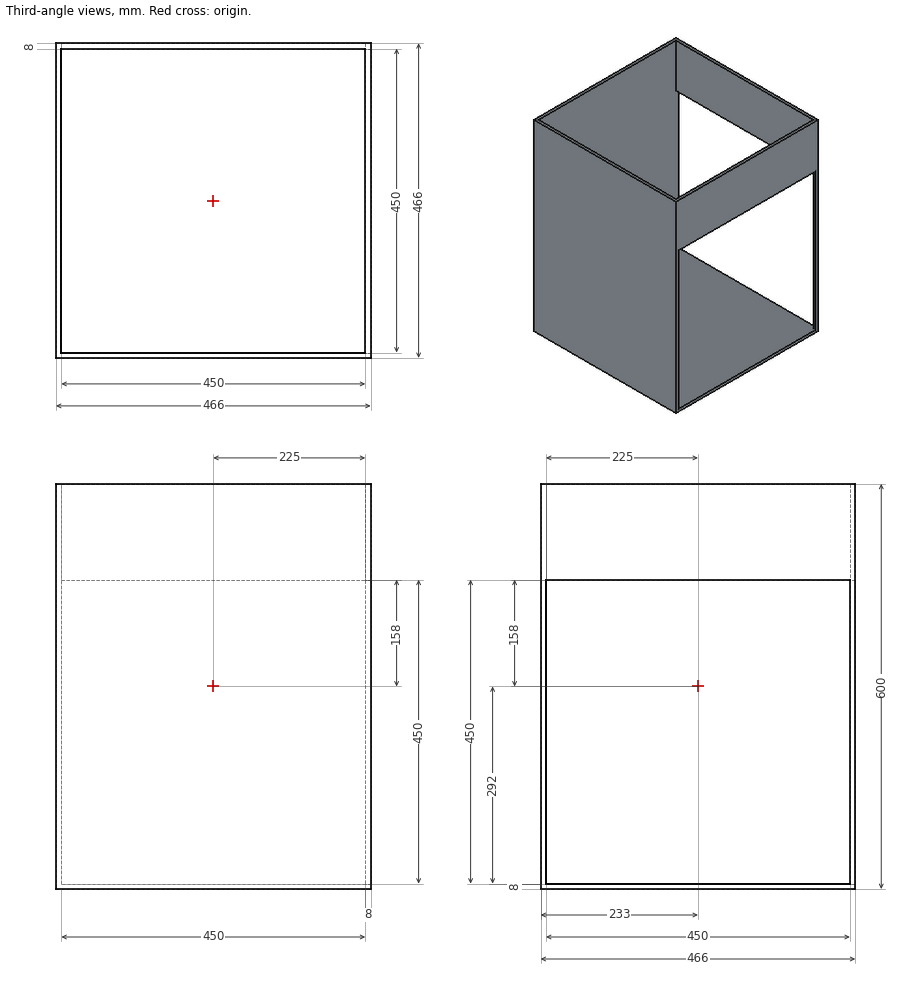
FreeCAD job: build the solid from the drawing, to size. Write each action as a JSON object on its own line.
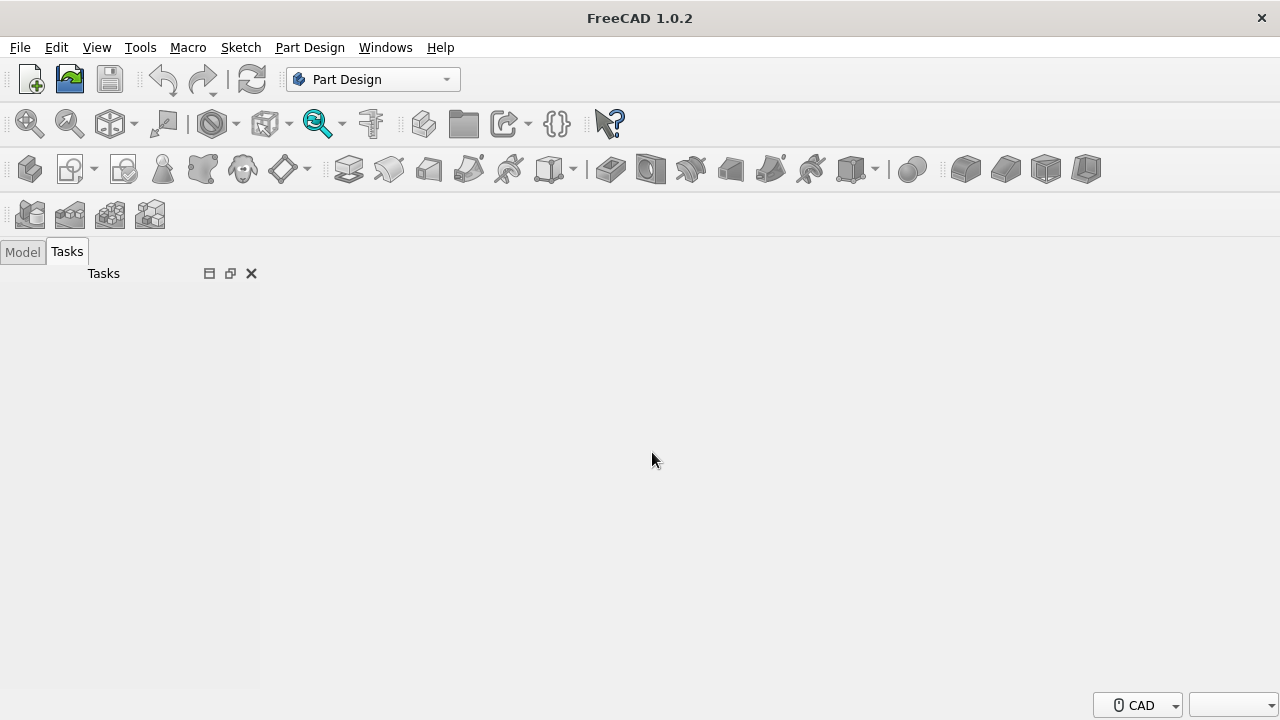
{"action": "left_click", "coordinate": [30, 80]}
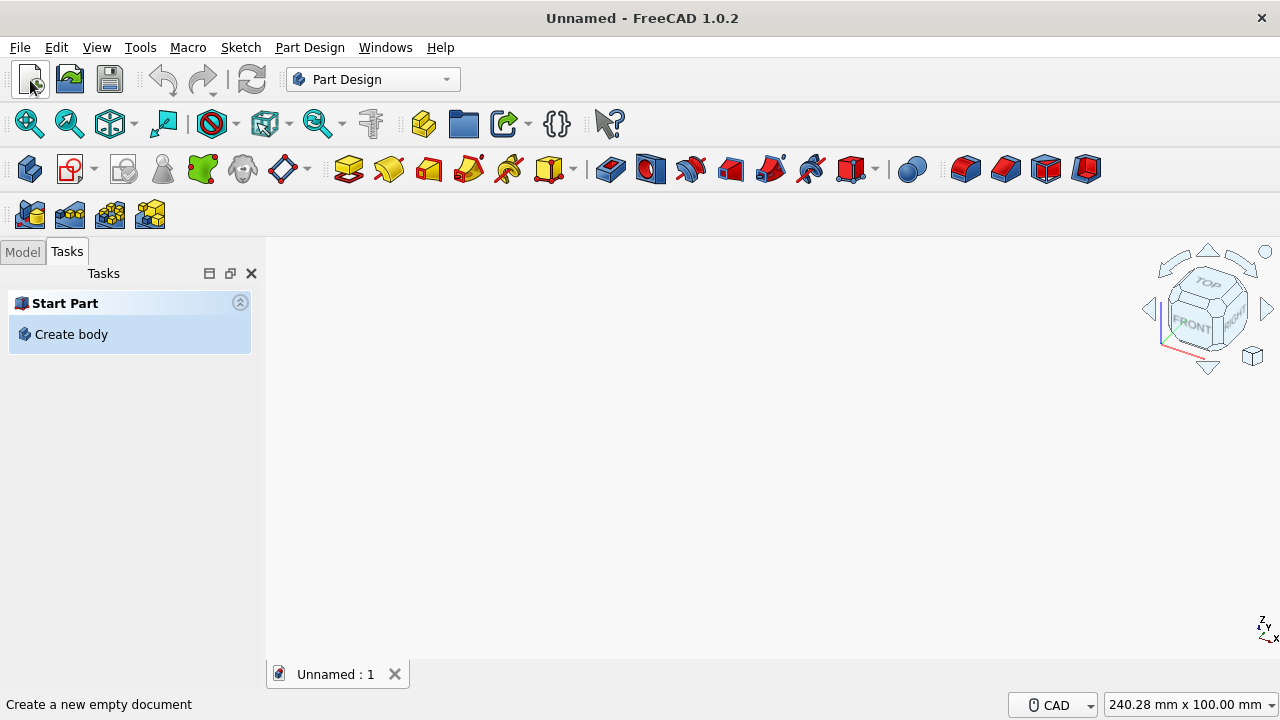
{"action": "left_click", "coordinate": [70, 170]}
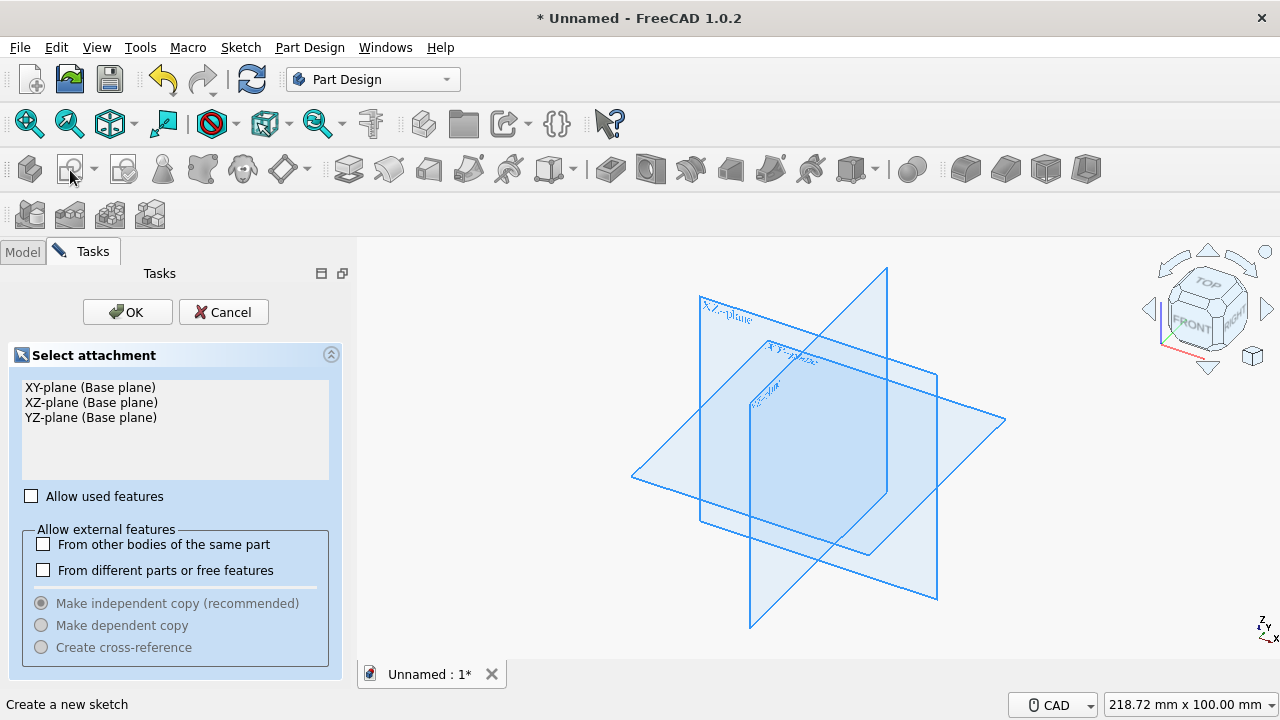
{"action": "left_click", "coordinate": [82, 388]}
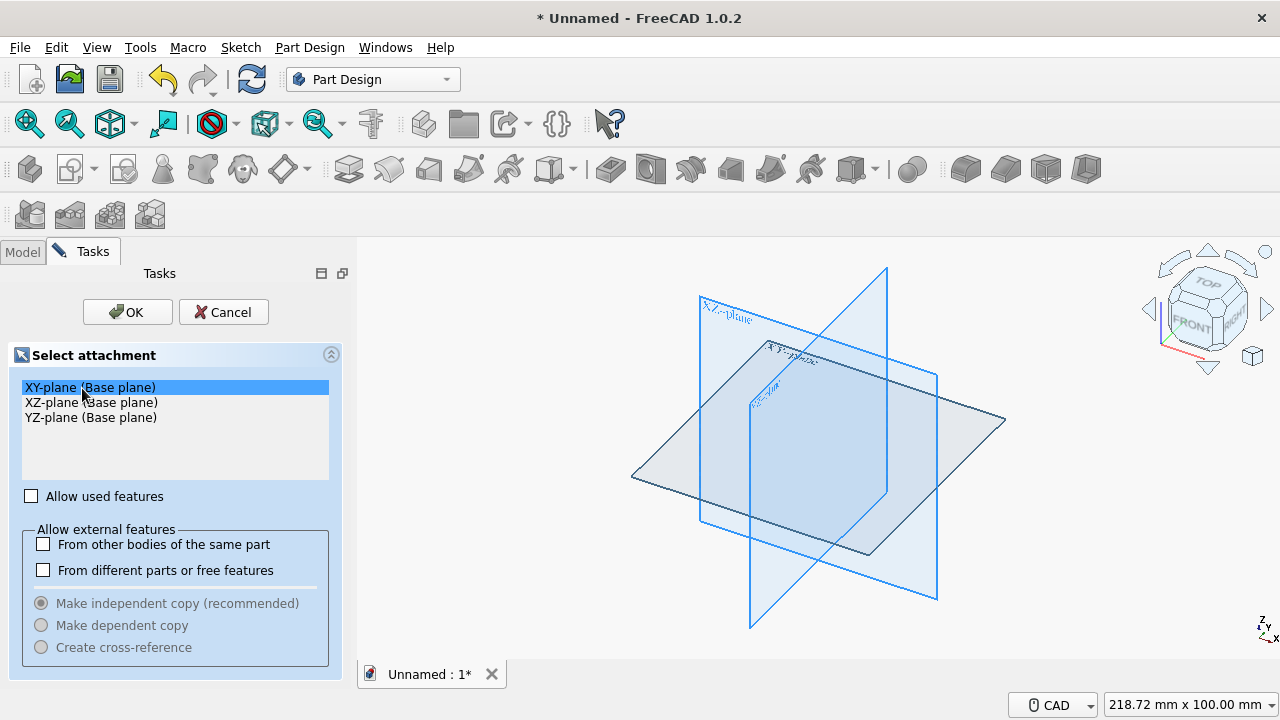
{"action": "left_click", "coordinate": [128, 312]}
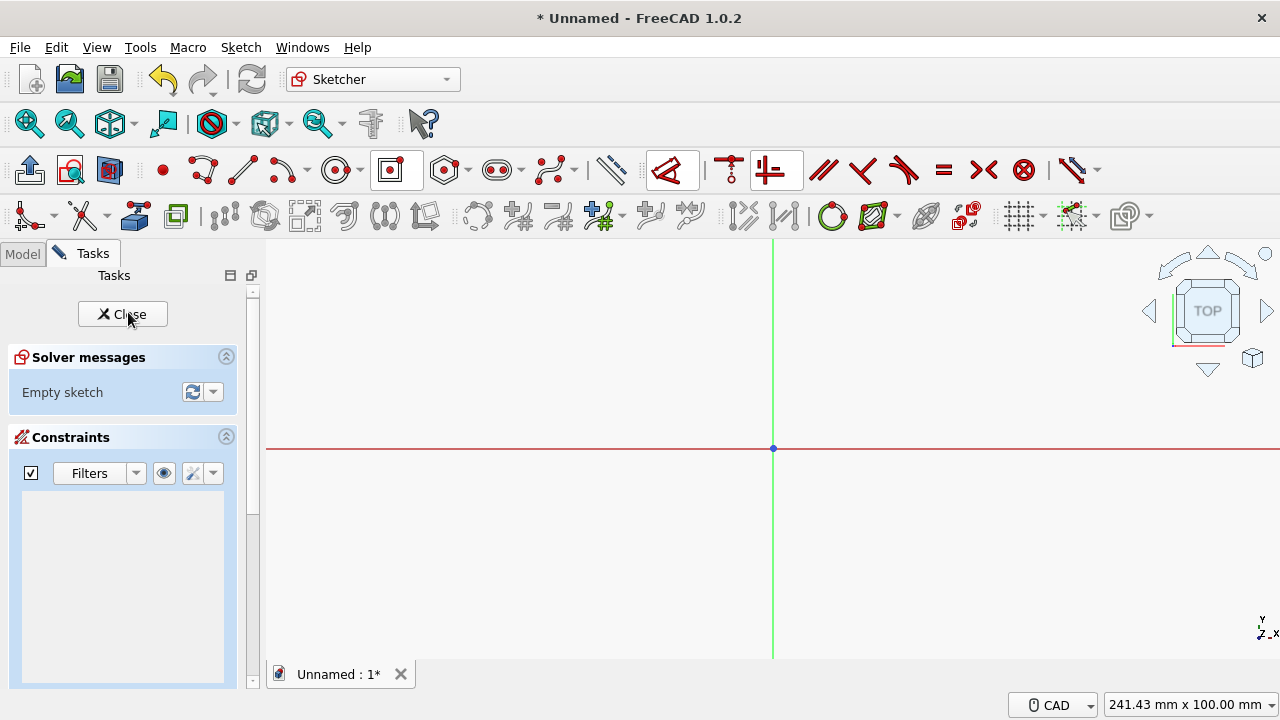
{"action": "scroll", "coordinate": [694, 449], "scroll_direction": "down", "scroll_amount": 10}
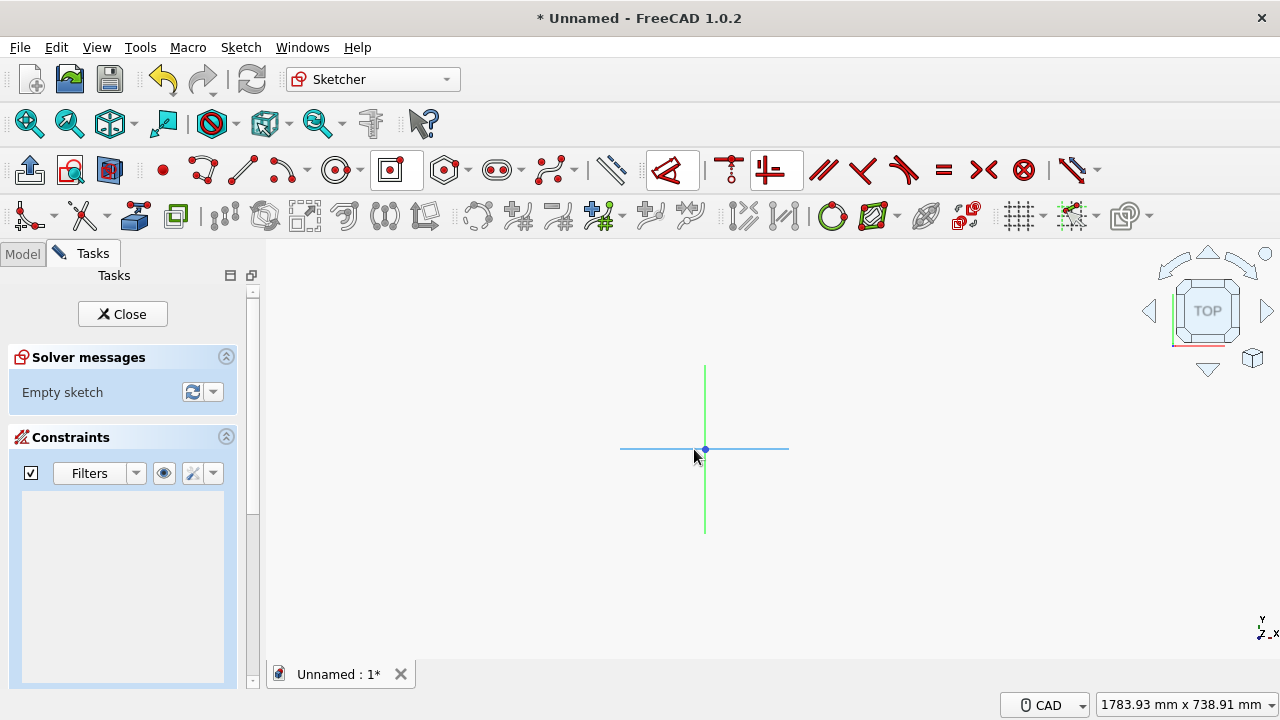
{"action": "left_click", "coordinate": [390, 170]}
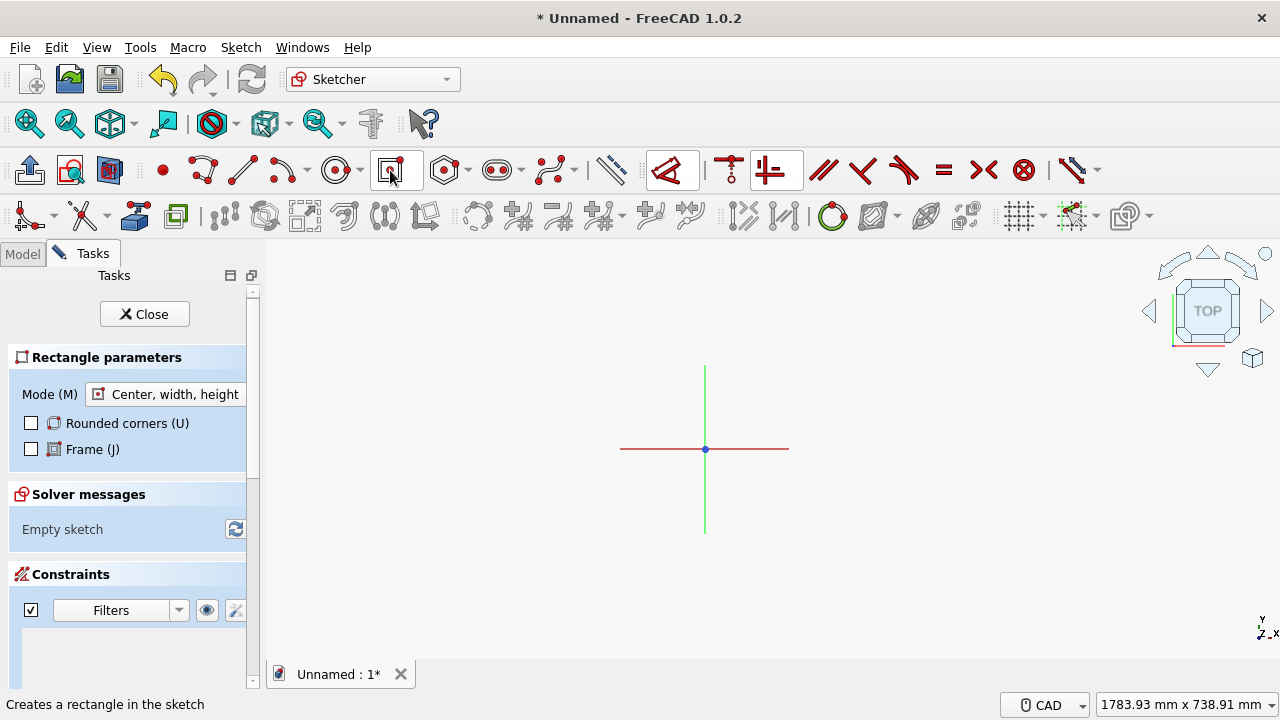
{"action": "left_click", "coordinate": [705, 449]}
{"action": "left_click", "coordinate": [837, 317]}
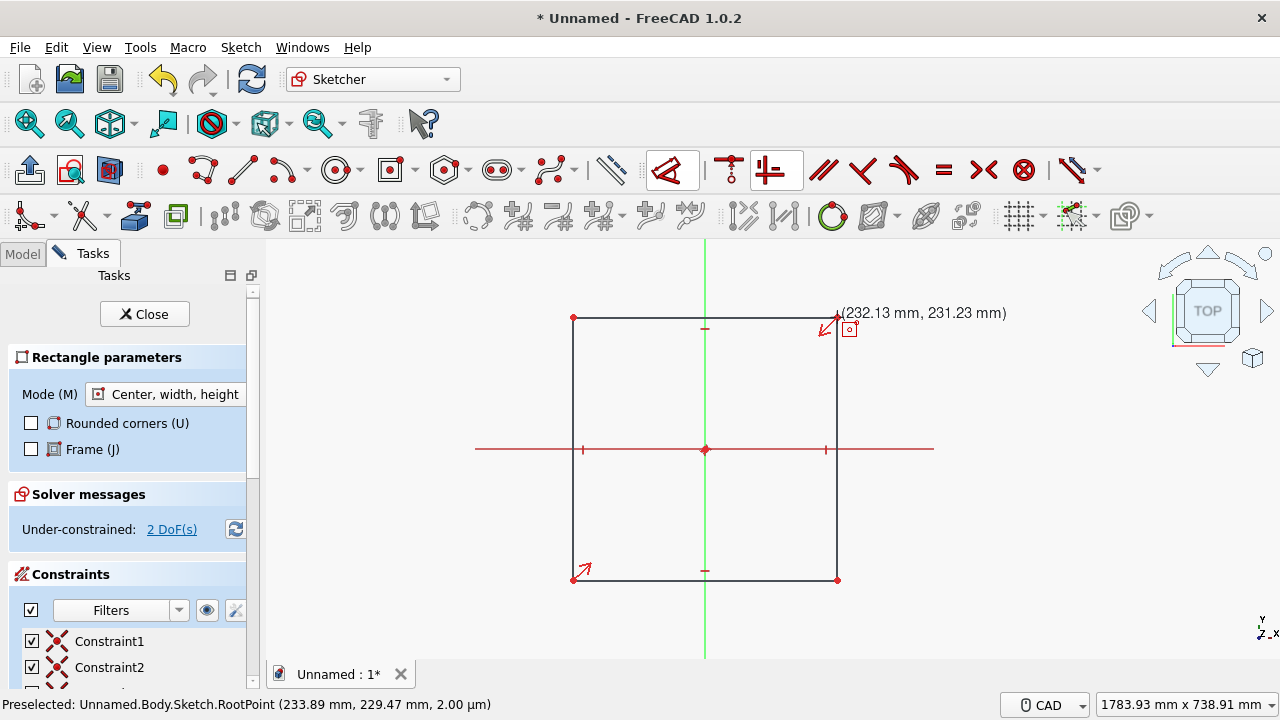
{"action": "left_click", "coordinate": [705, 449]}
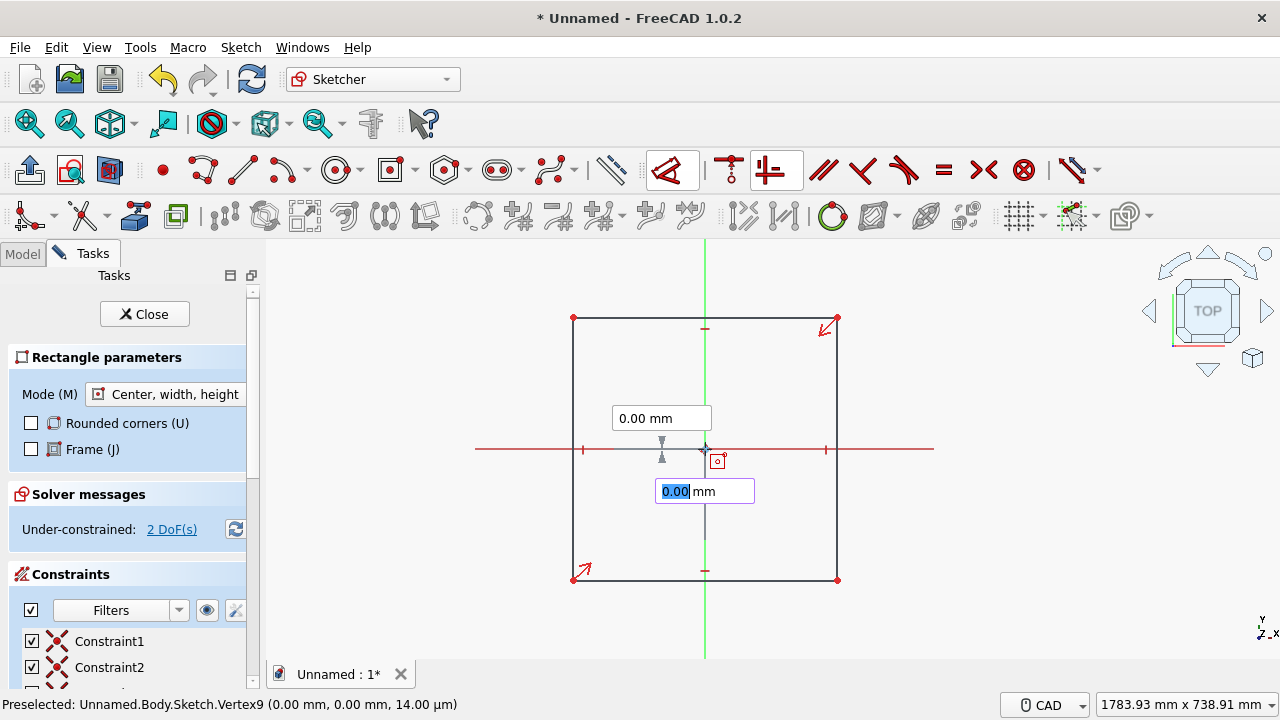
{"action": "scroll", "coordinate": [833, 322], "scroll_direction": "up", "scroll_amount": 7}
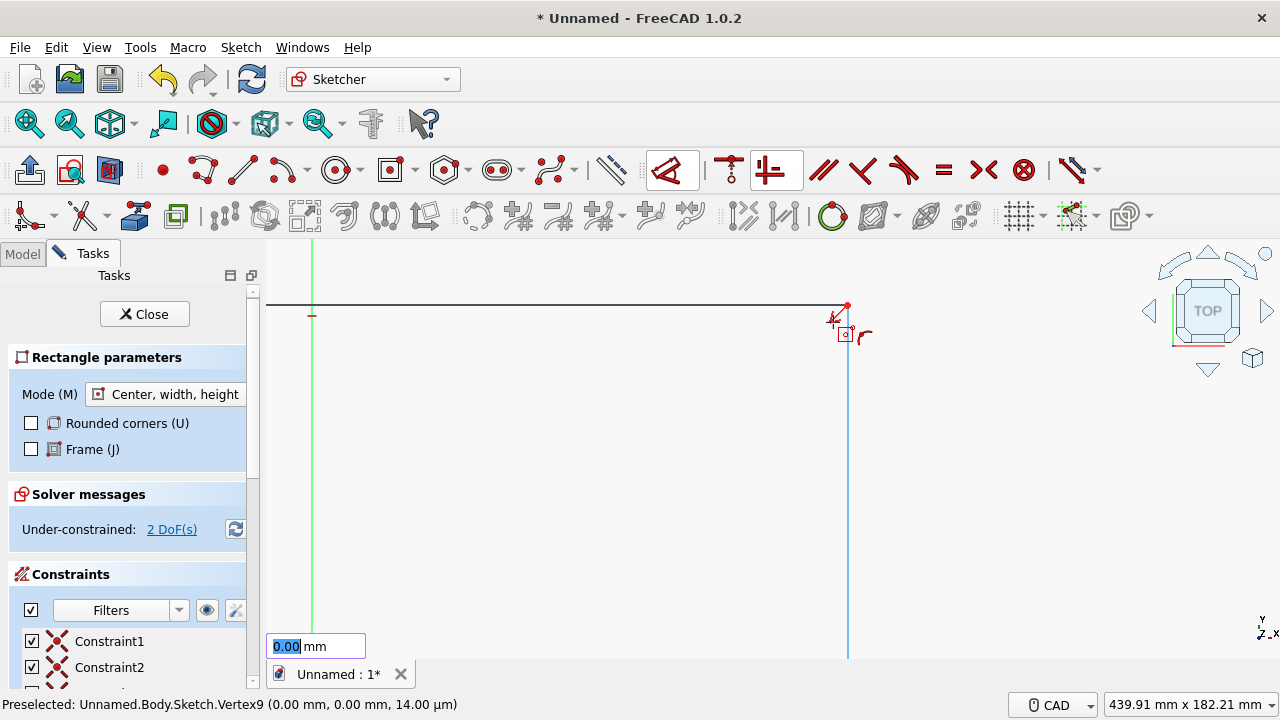
{"action": "left_click", "coordinate": [831, 320]}
{"action": "key", "text": "Escape"}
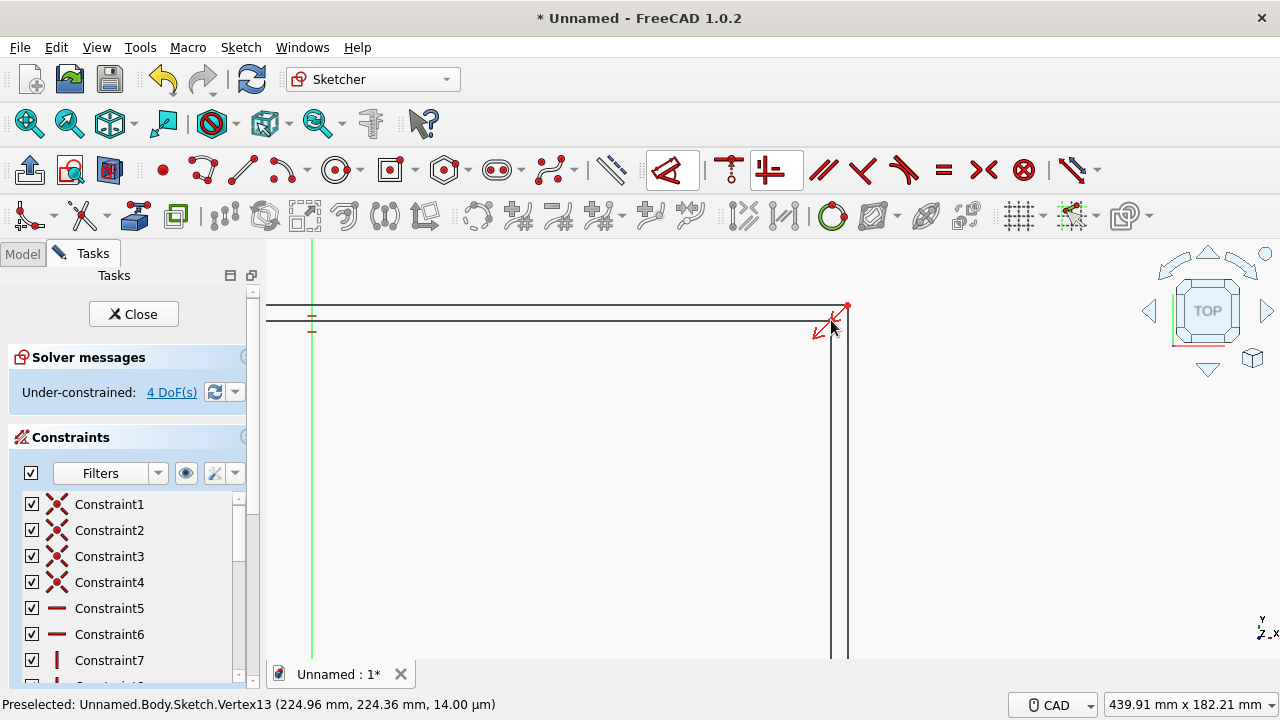
{"action": "scroll", "coordinate": [833, 322], "scroll_direction": "down", "scroll_amount": 7}